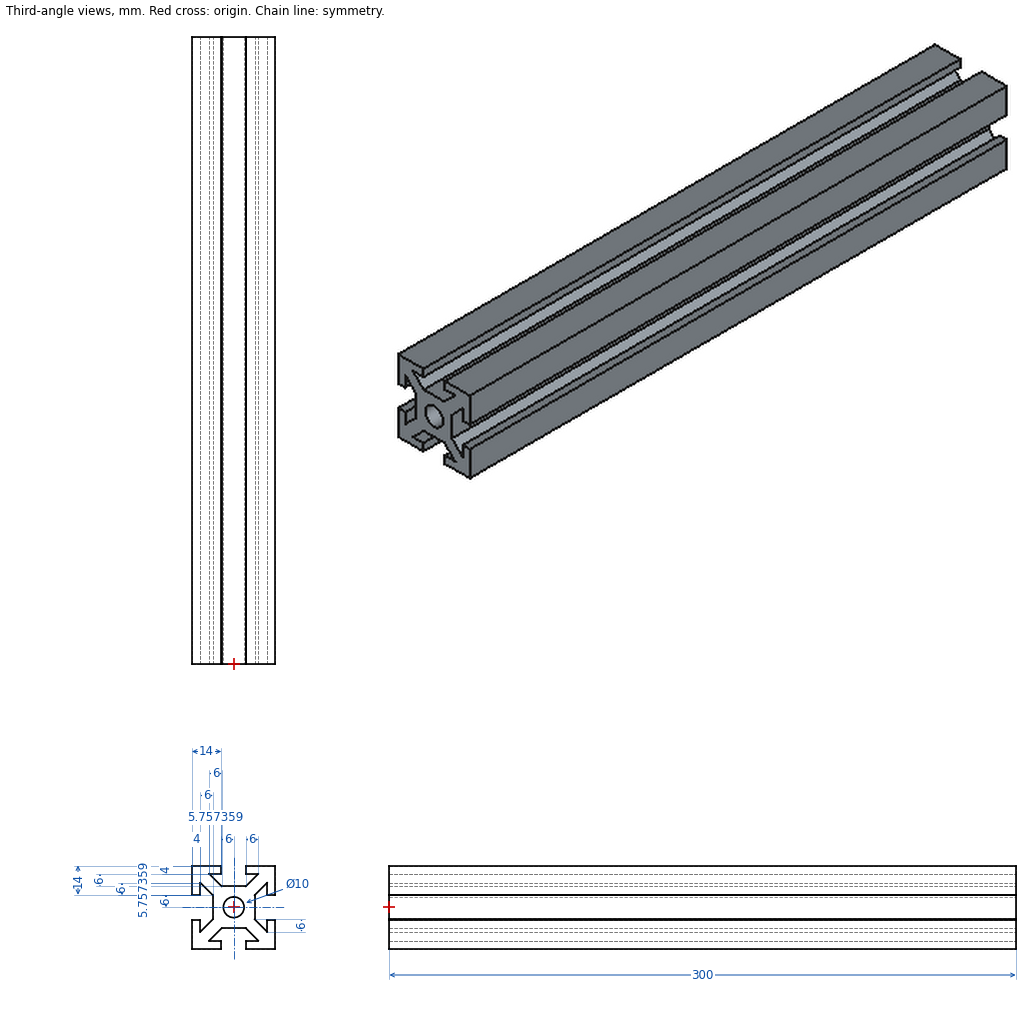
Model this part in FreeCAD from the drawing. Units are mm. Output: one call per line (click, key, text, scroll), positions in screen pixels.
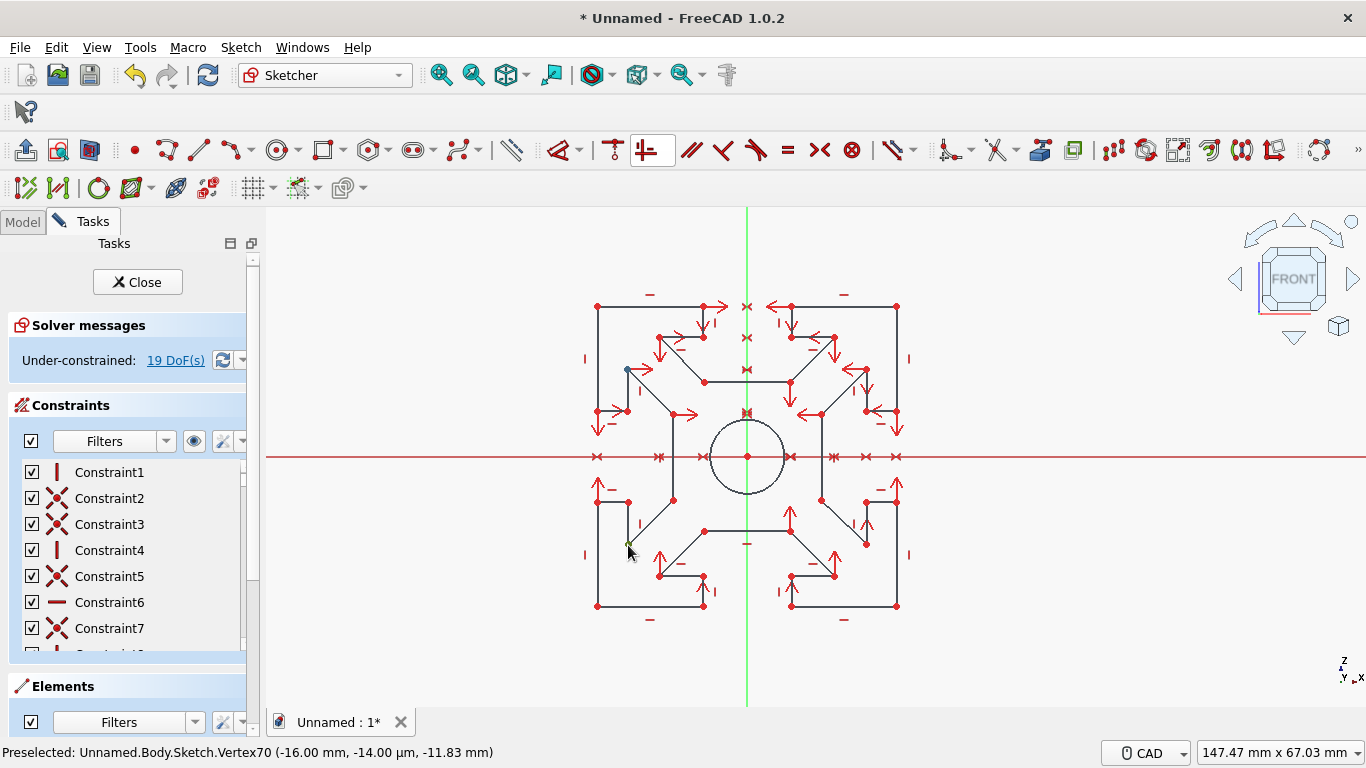
click(359, 457)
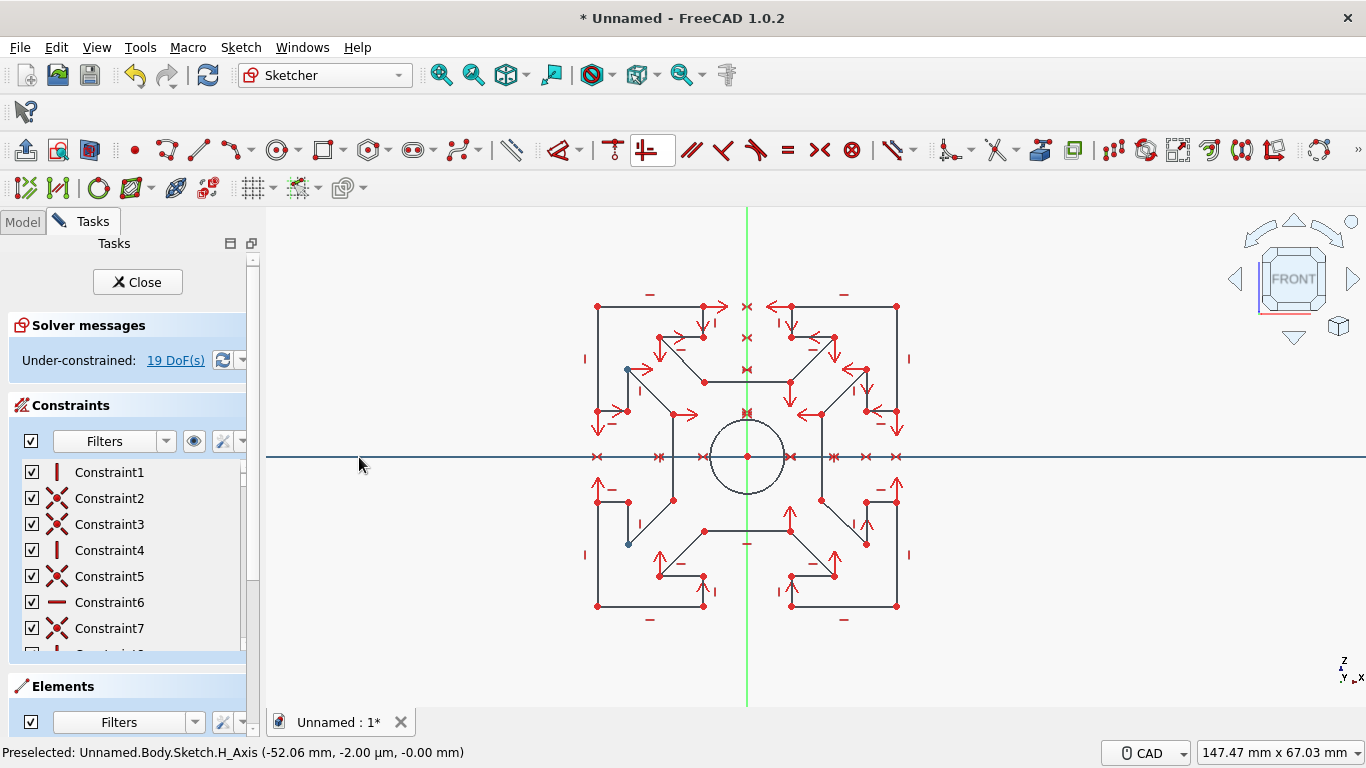
click(820, 150)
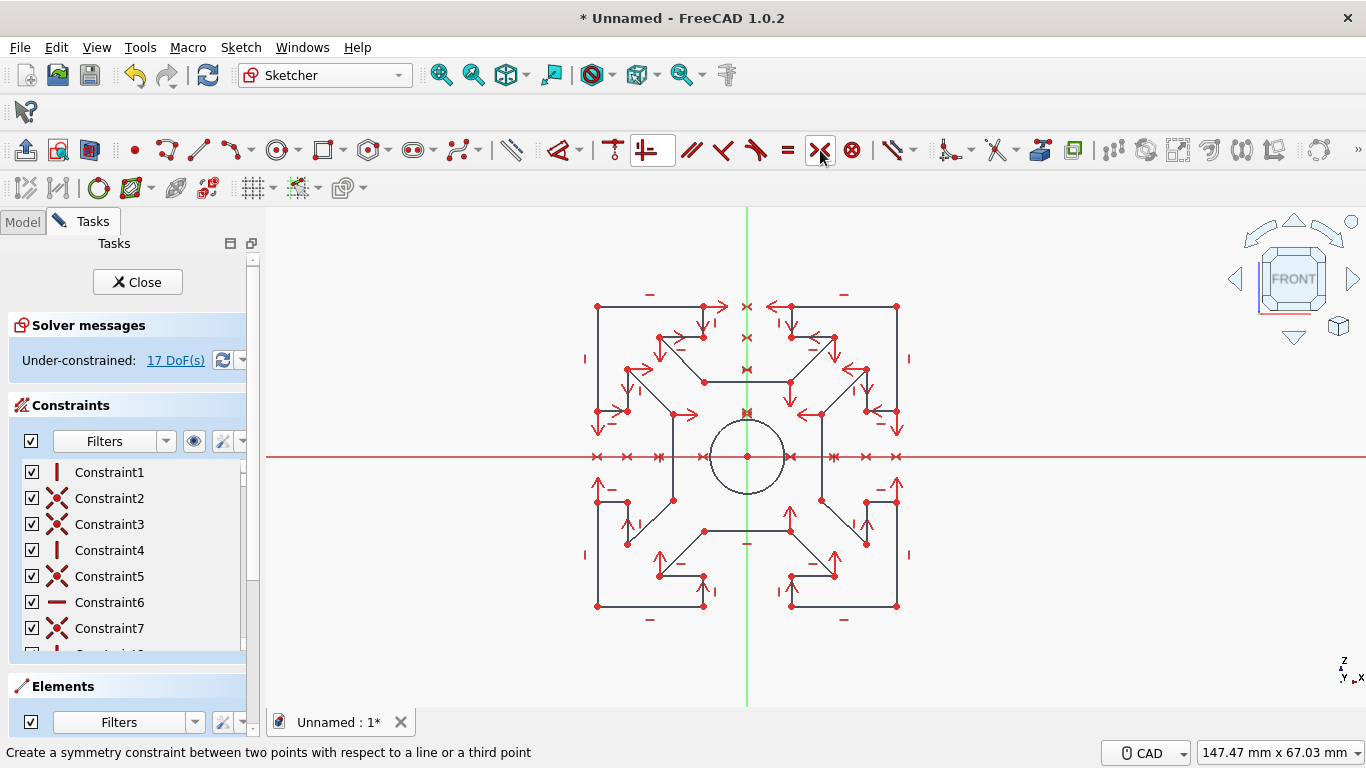
click(558, 150)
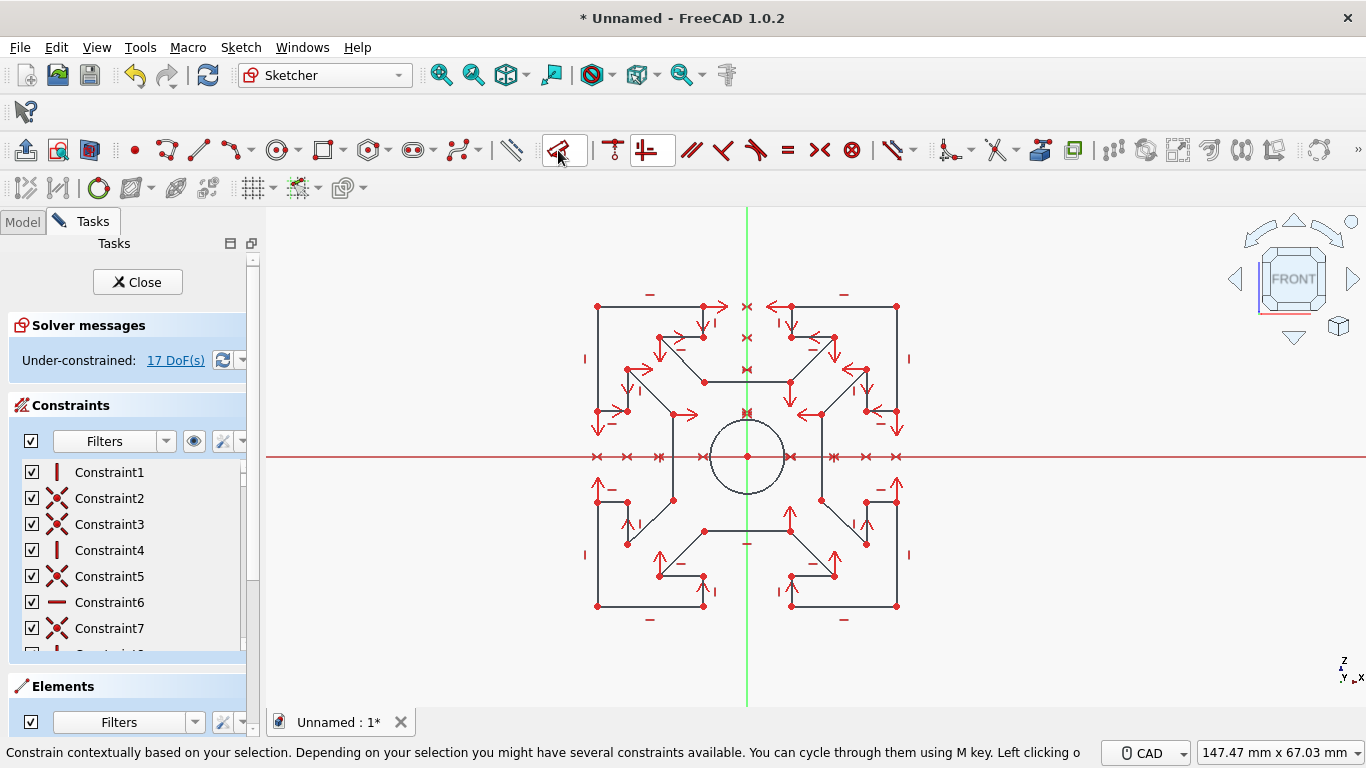
click(773, 430)
click(795, 407)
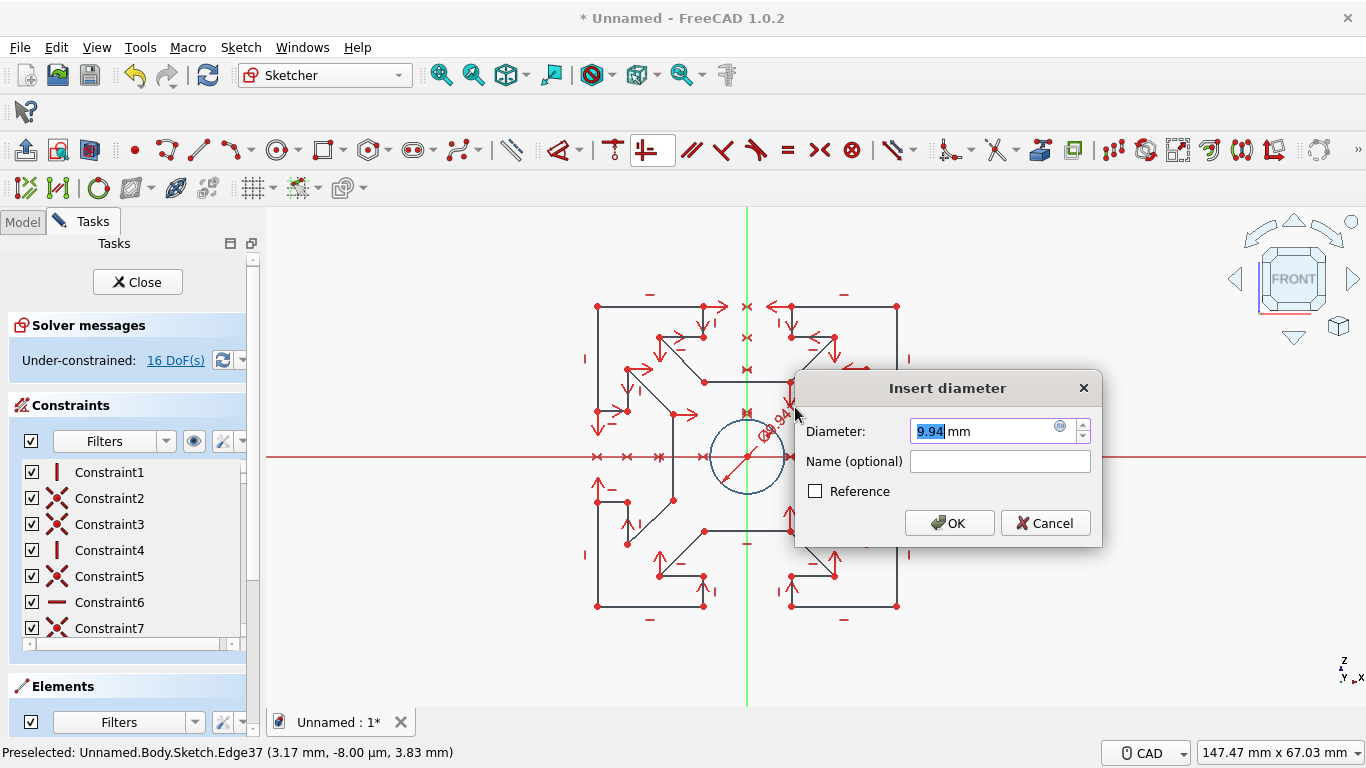
text(10)
key(Return)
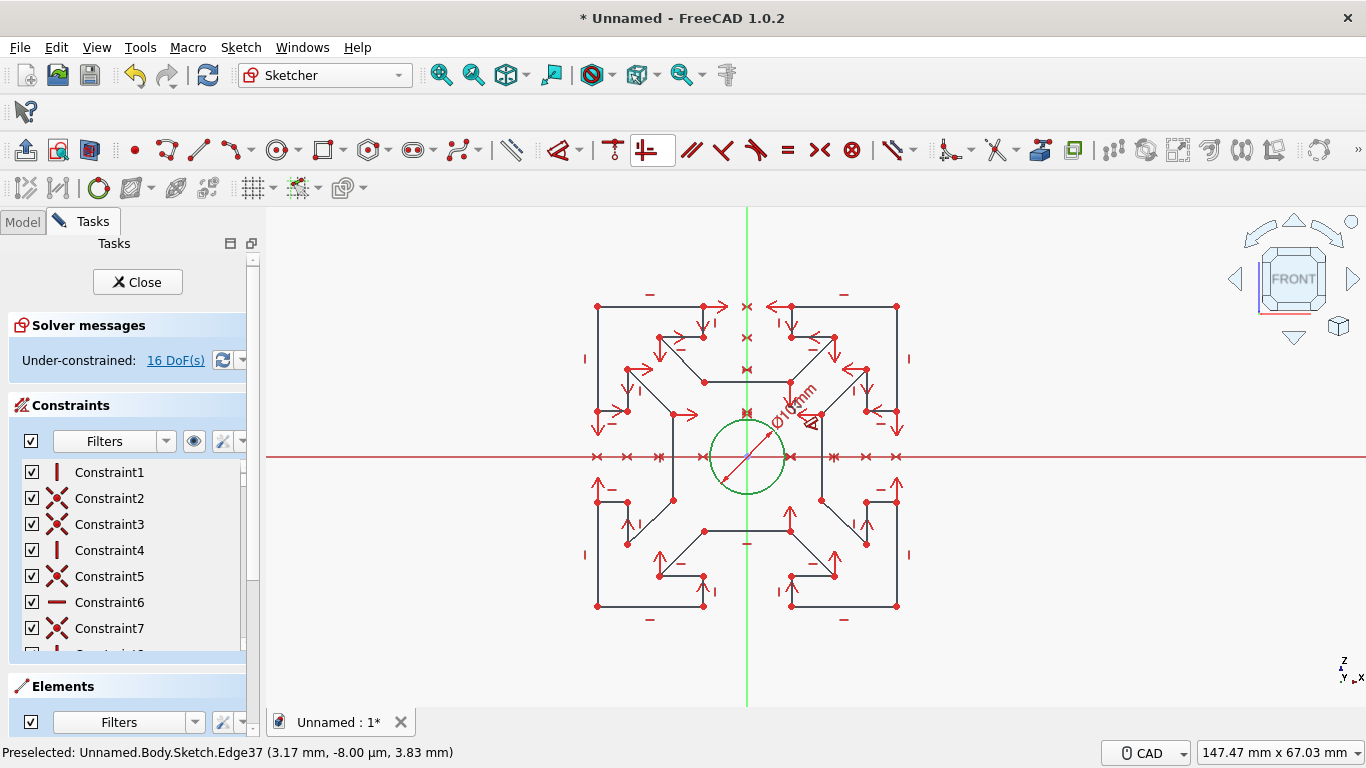
scroll(616, 411, up, 2)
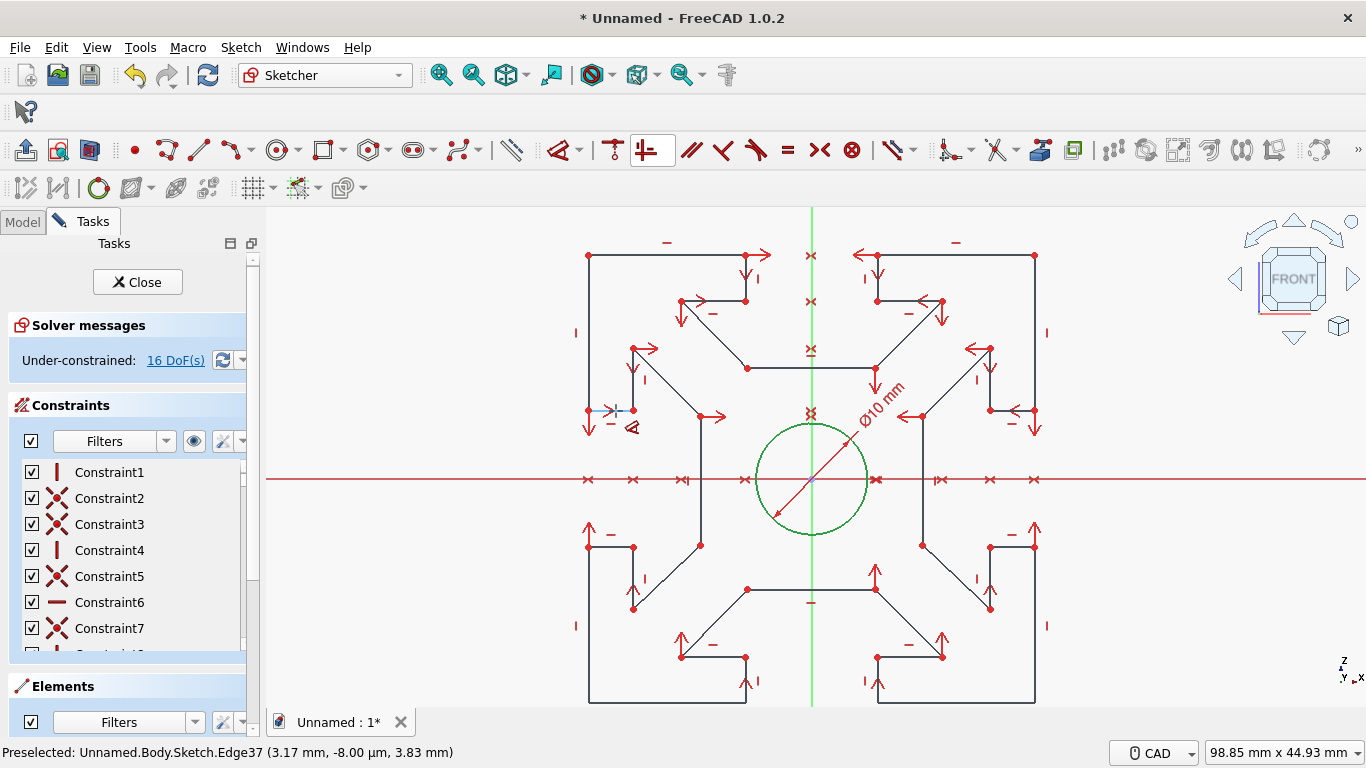
click(616, 411)
click(611, 377)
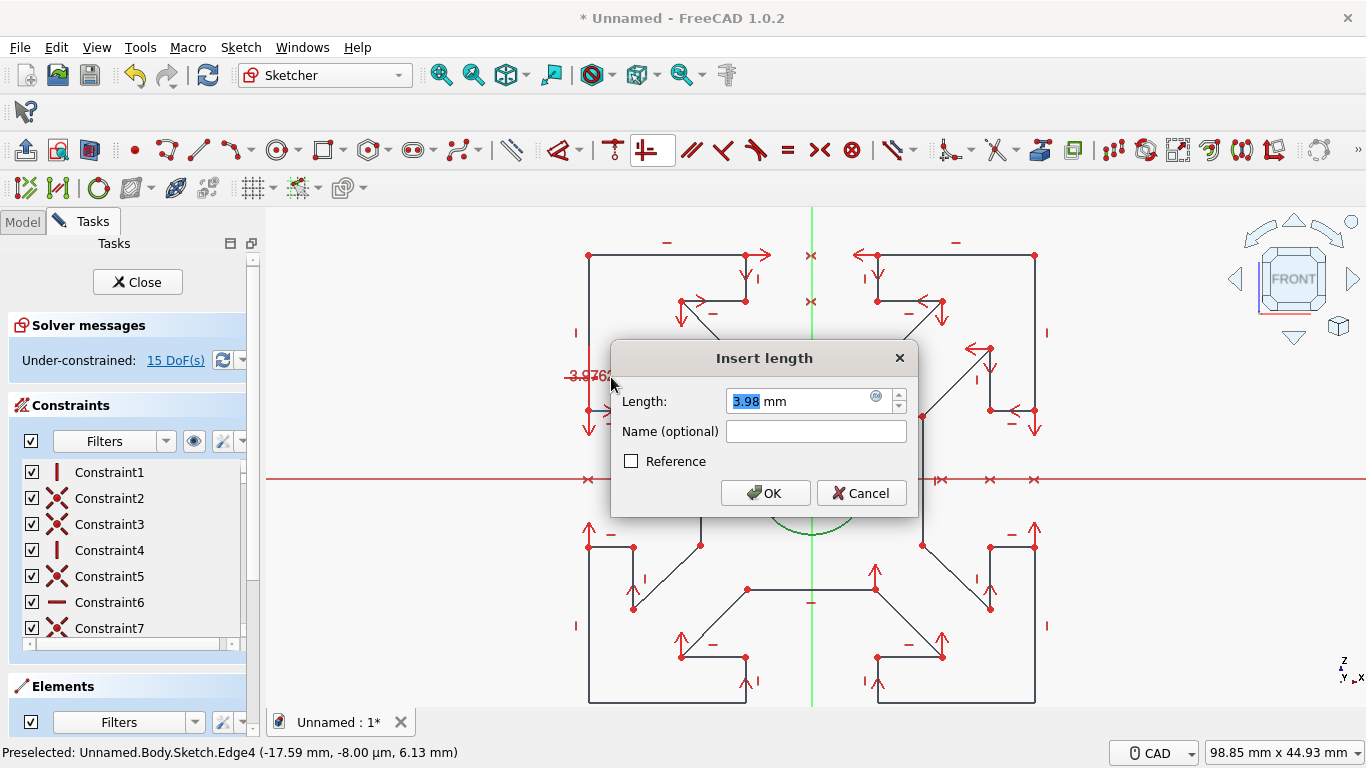
text(4)
key(Return)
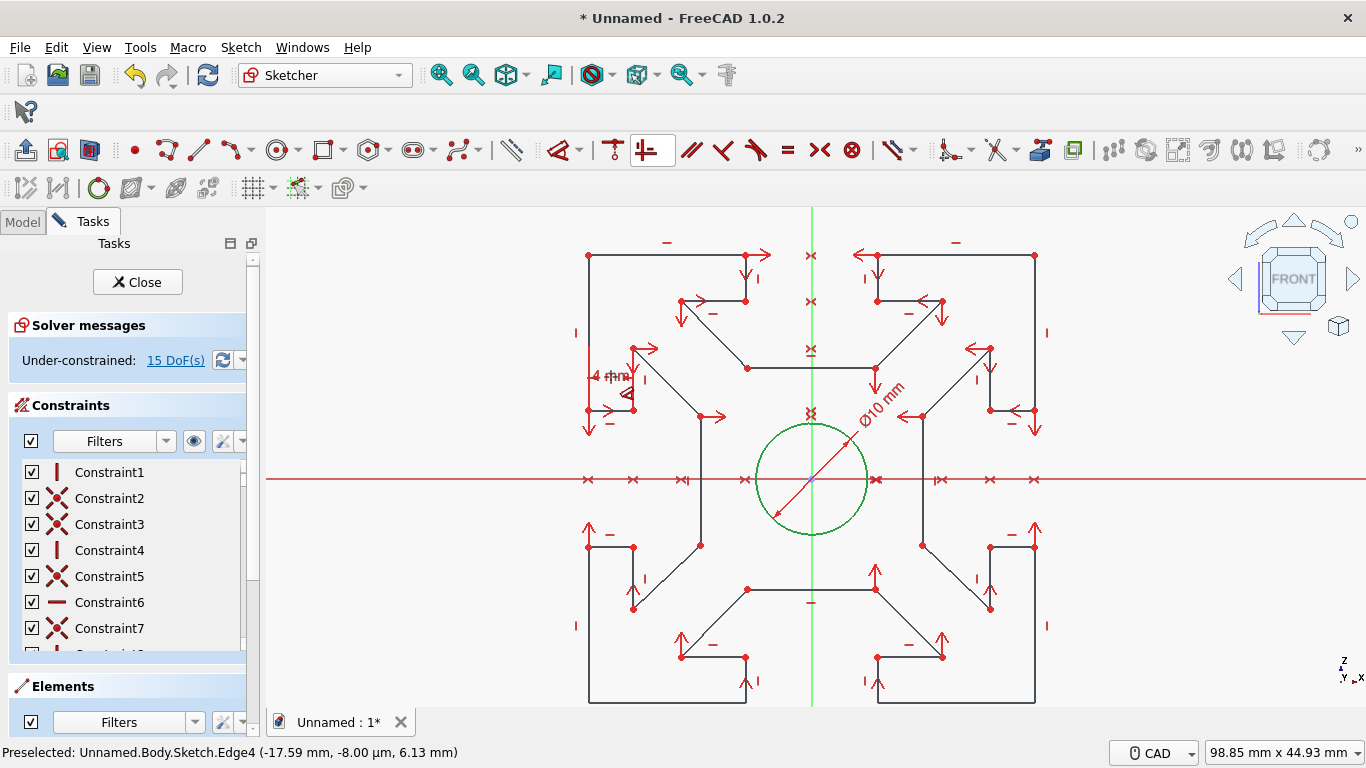
click(746, 269)
click(712, 278)